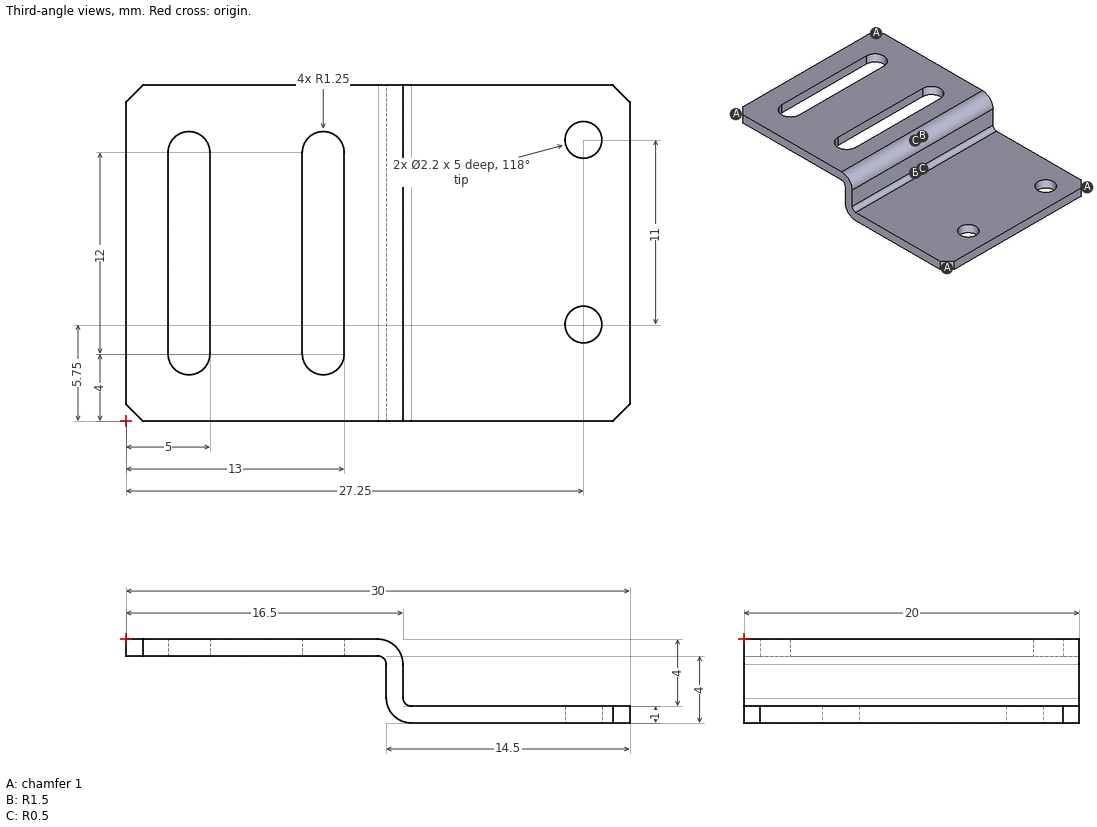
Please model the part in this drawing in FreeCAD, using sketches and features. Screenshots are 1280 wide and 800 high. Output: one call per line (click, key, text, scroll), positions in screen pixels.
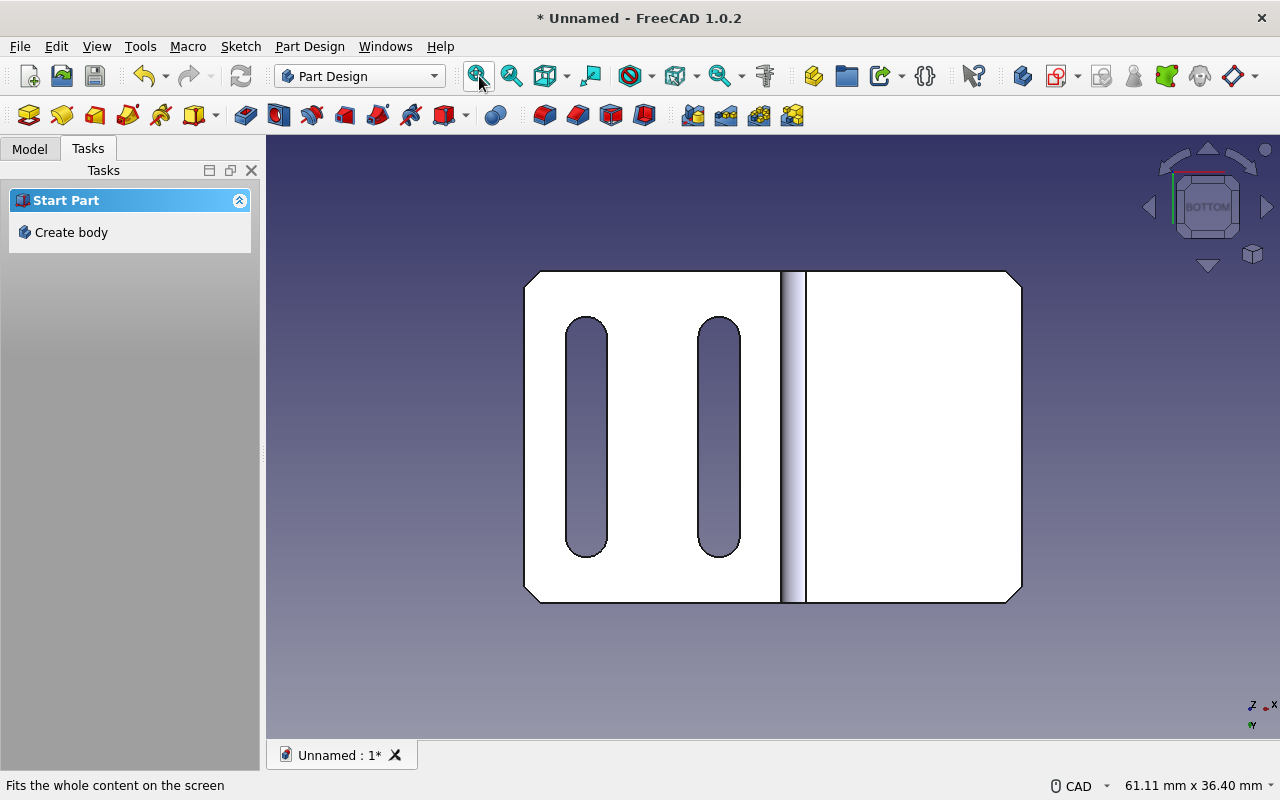
key(4)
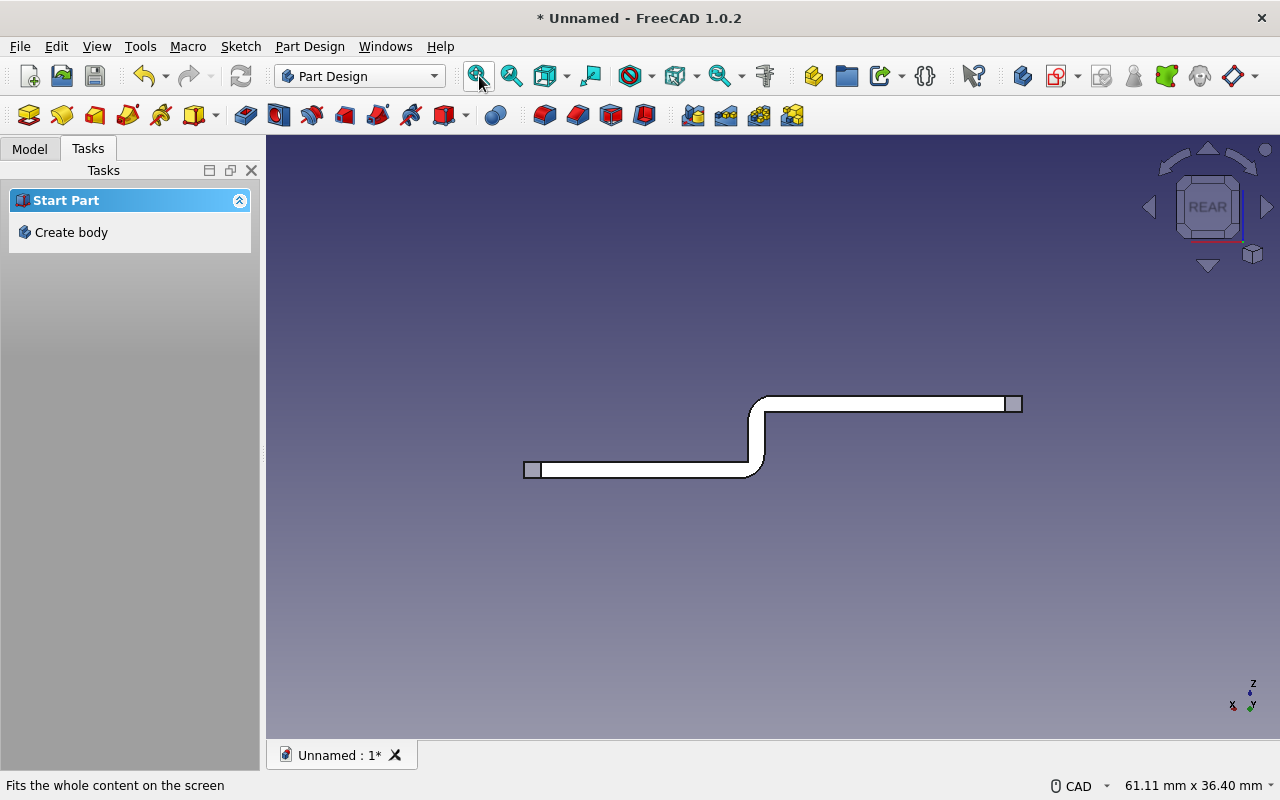
key(6)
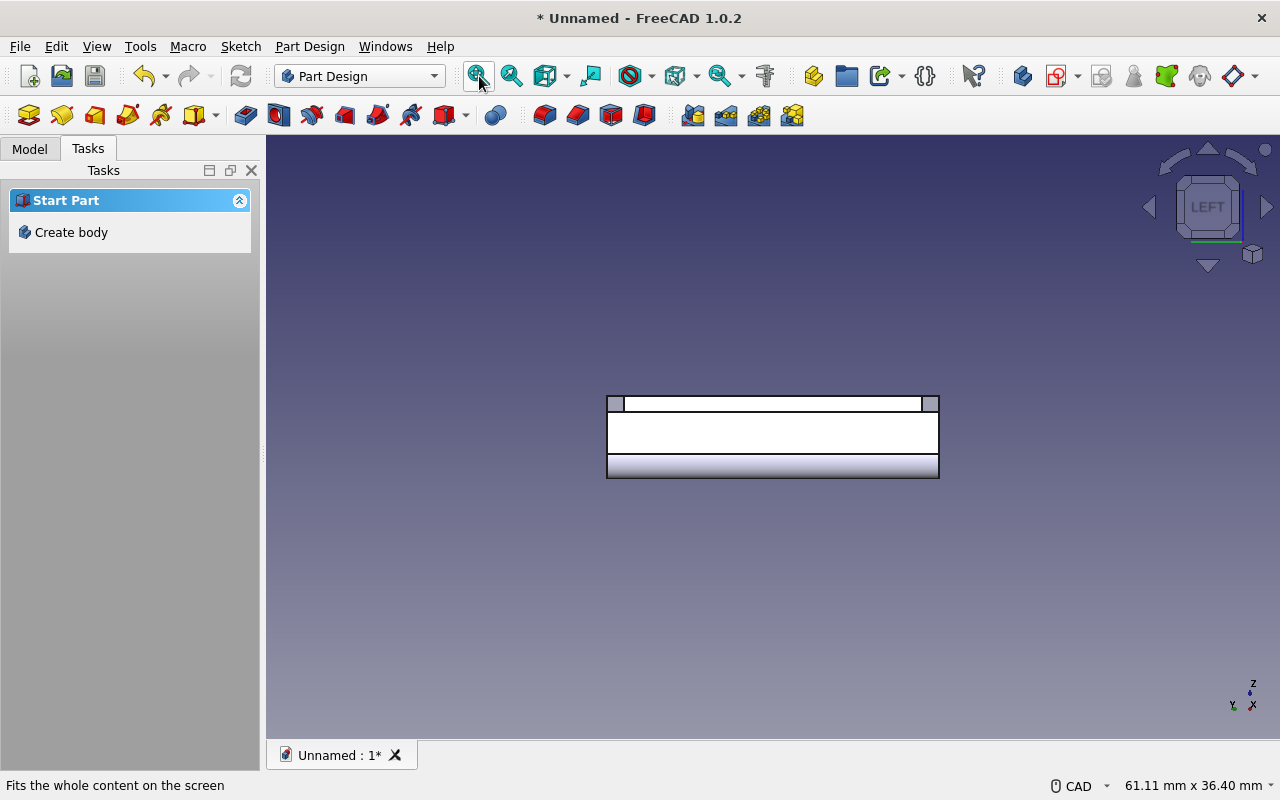
click(479, 76)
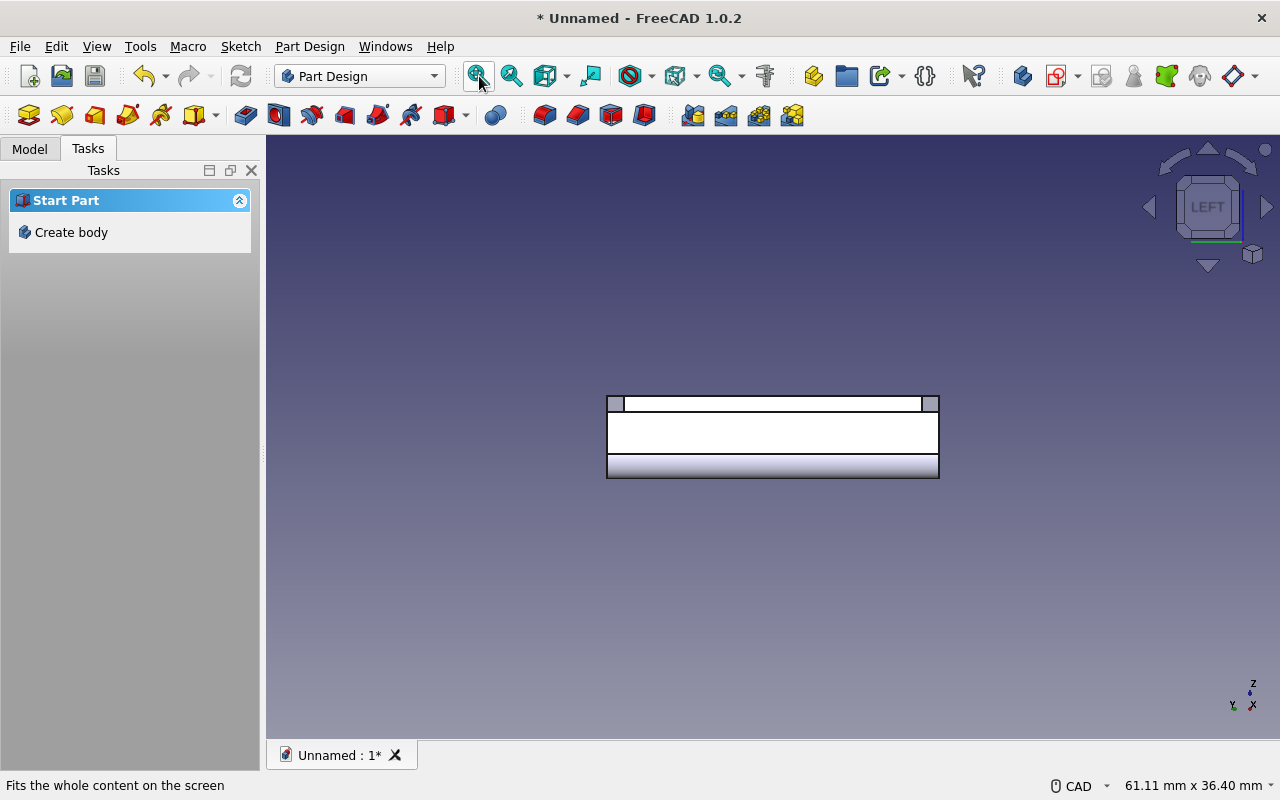
key(v)
key(3)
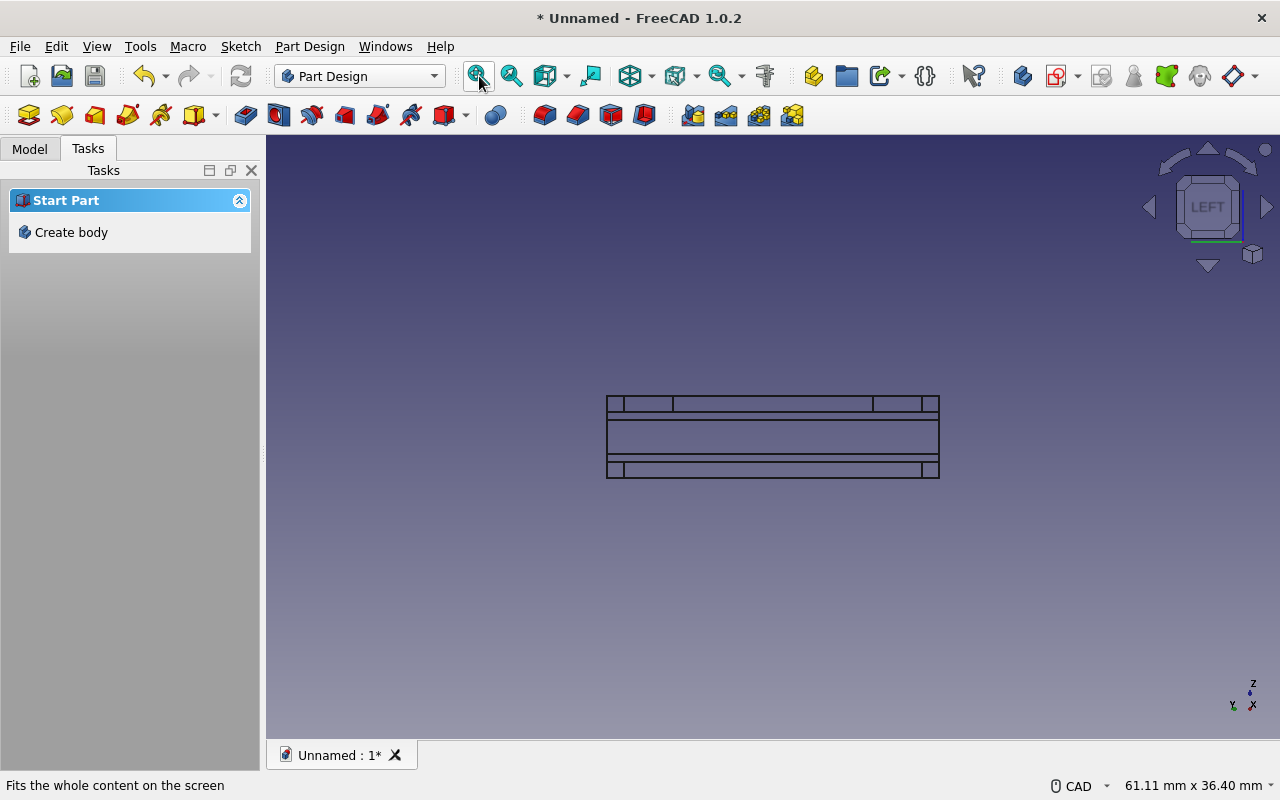
key(0)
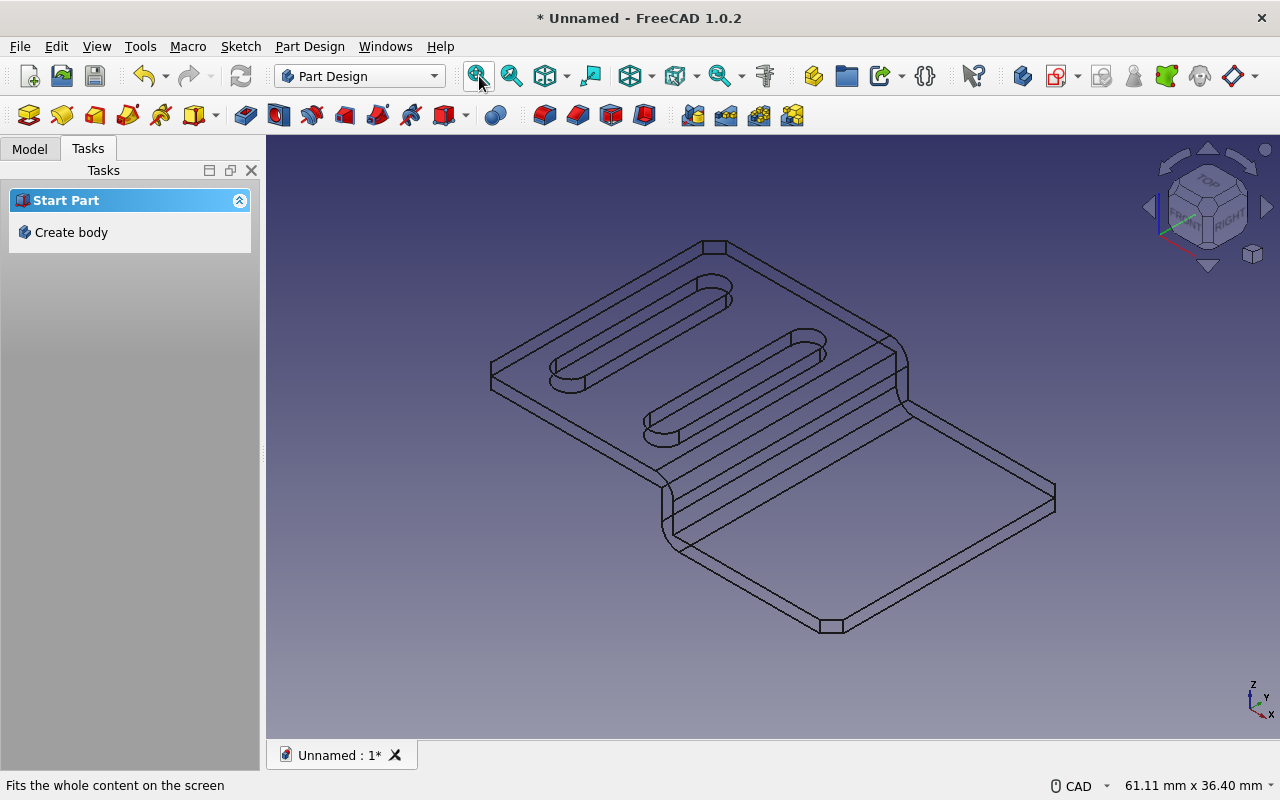
click(779, 419)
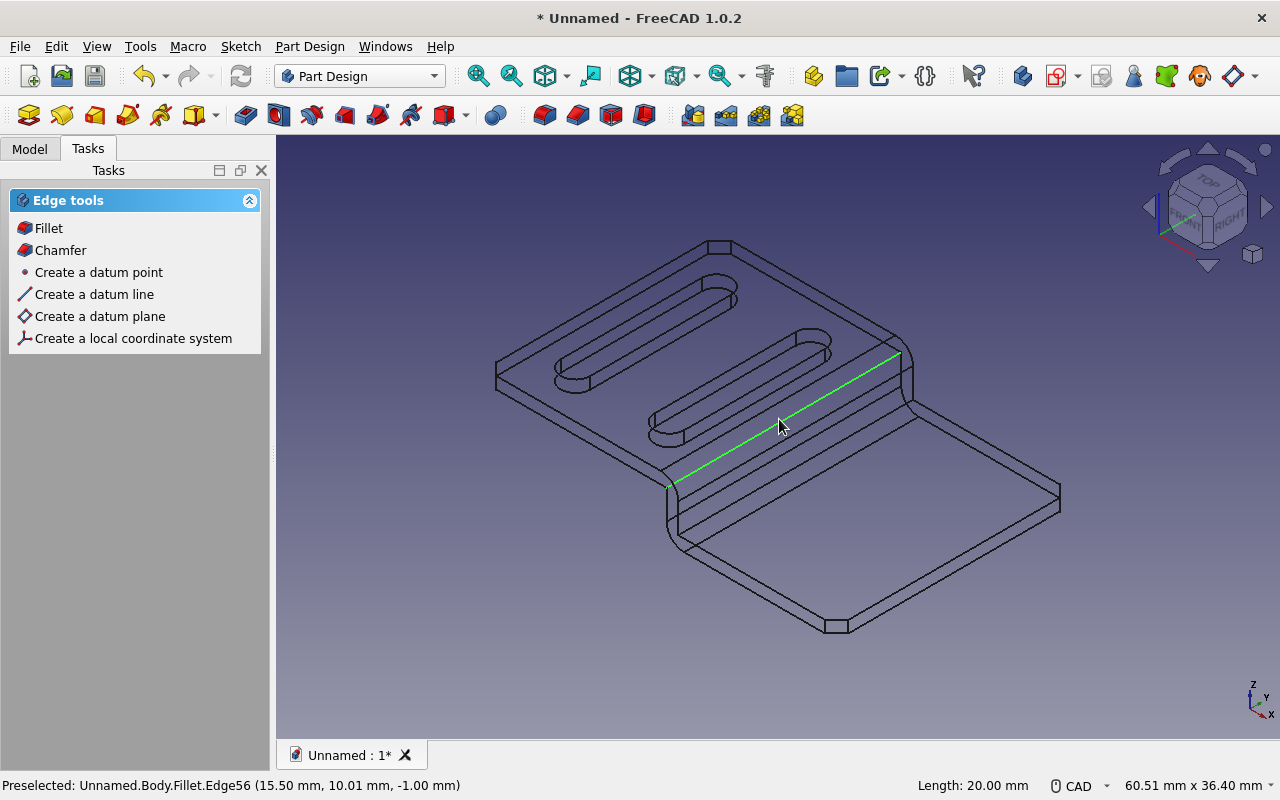
click(796, 466, ctrl)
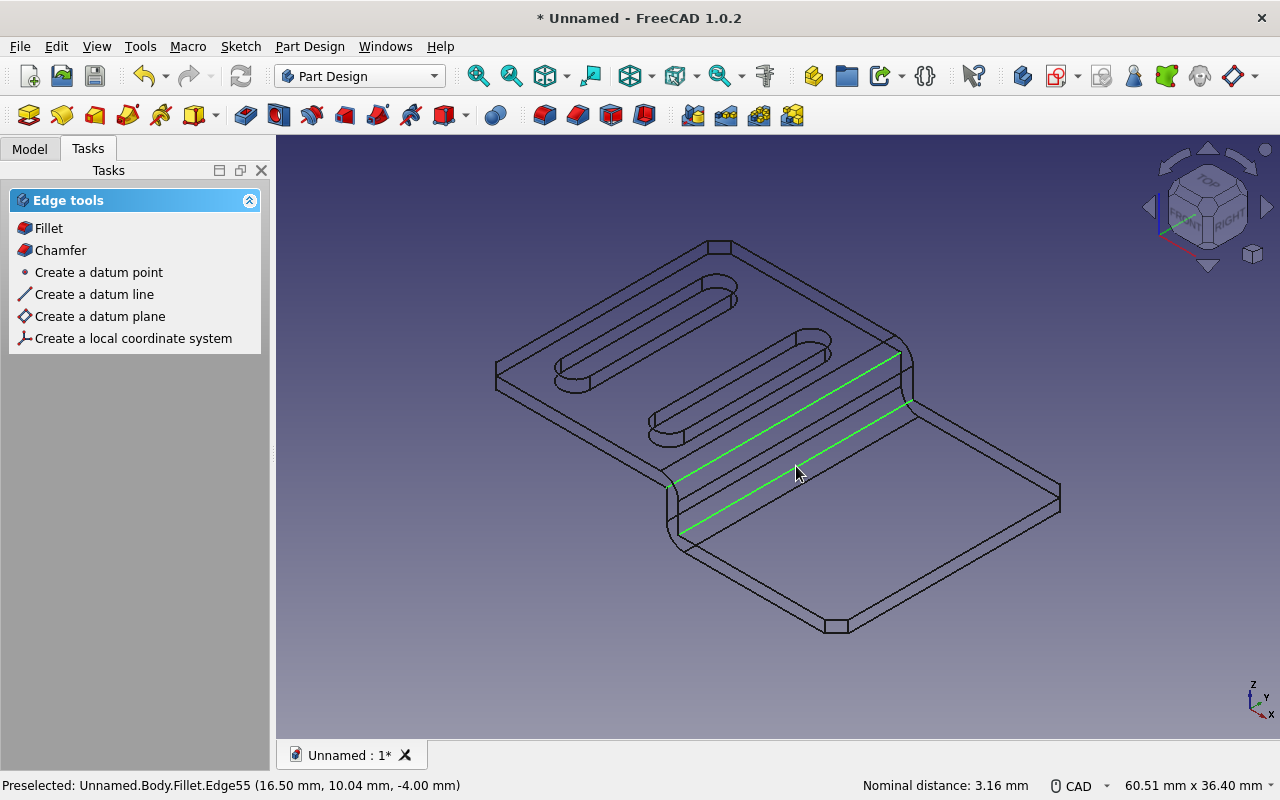
key(v)
key(1)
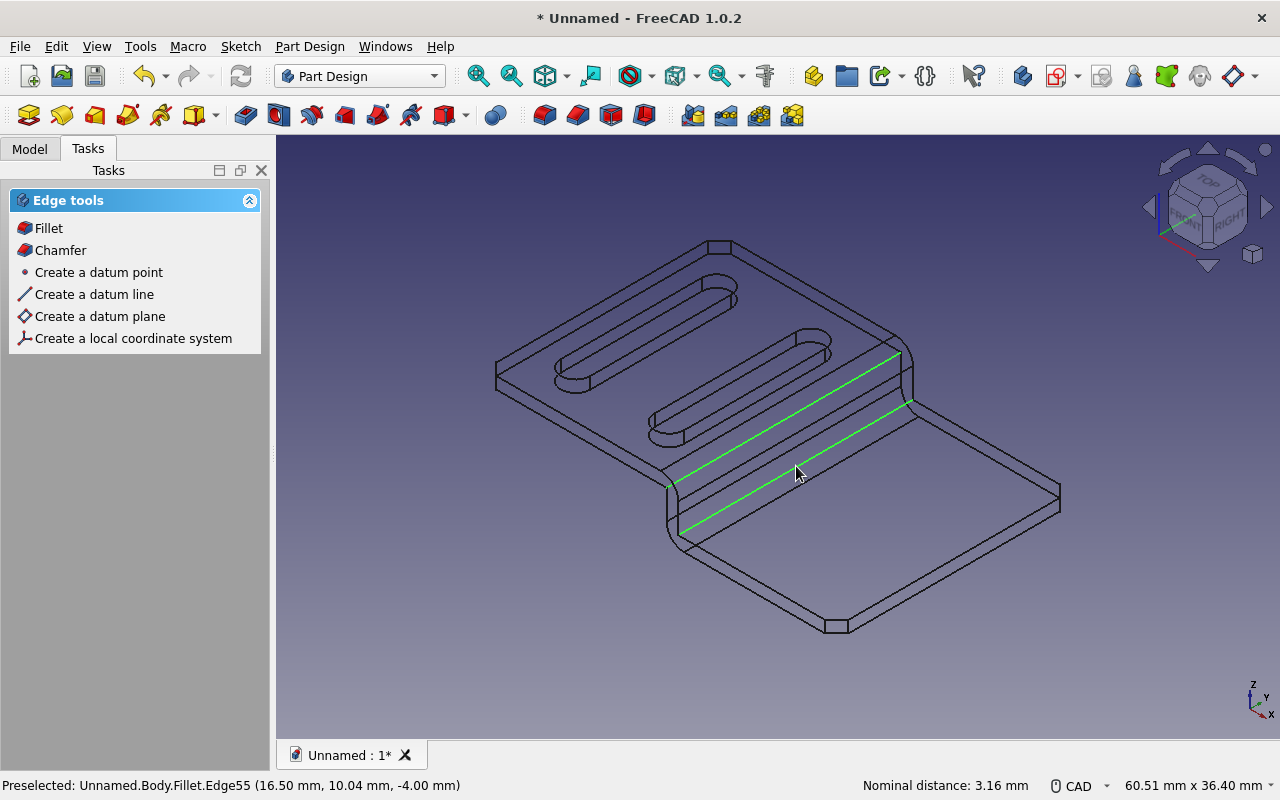
click(545, 116)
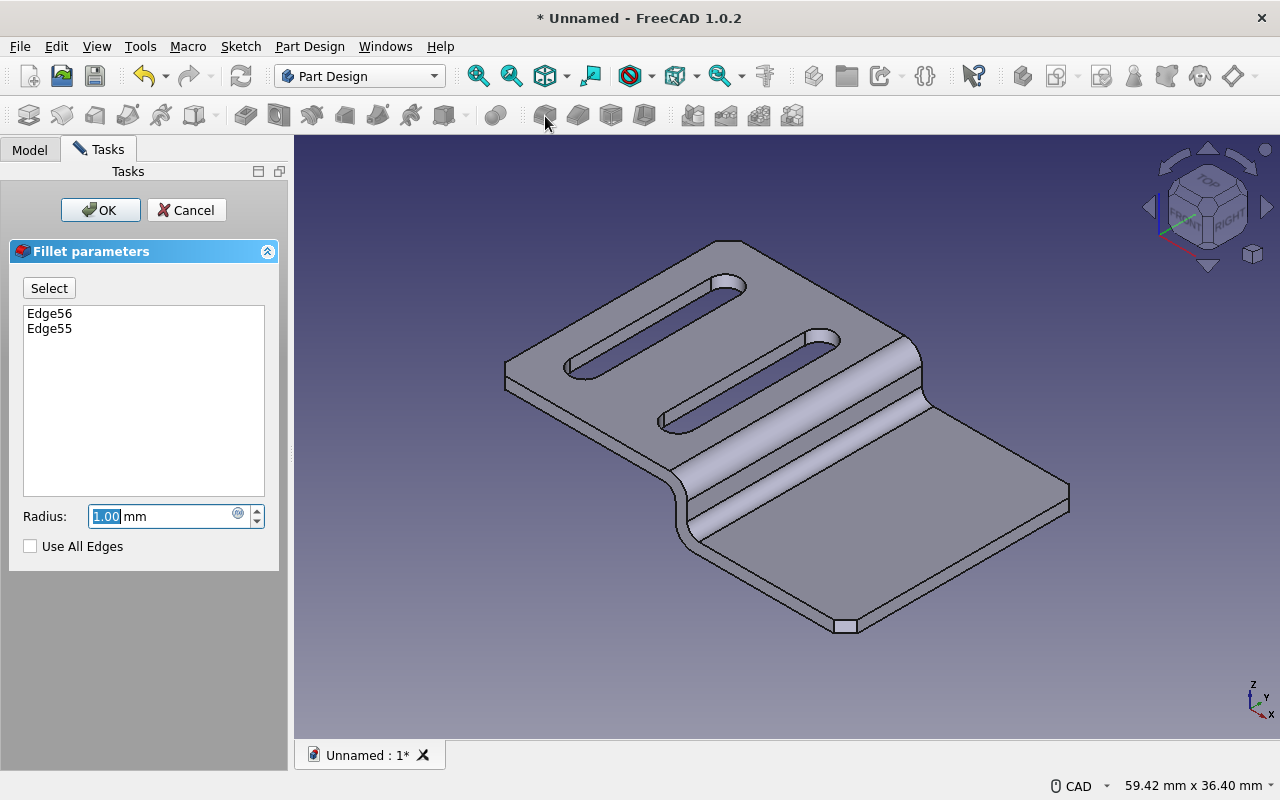
text(0.5)
key(Tab)